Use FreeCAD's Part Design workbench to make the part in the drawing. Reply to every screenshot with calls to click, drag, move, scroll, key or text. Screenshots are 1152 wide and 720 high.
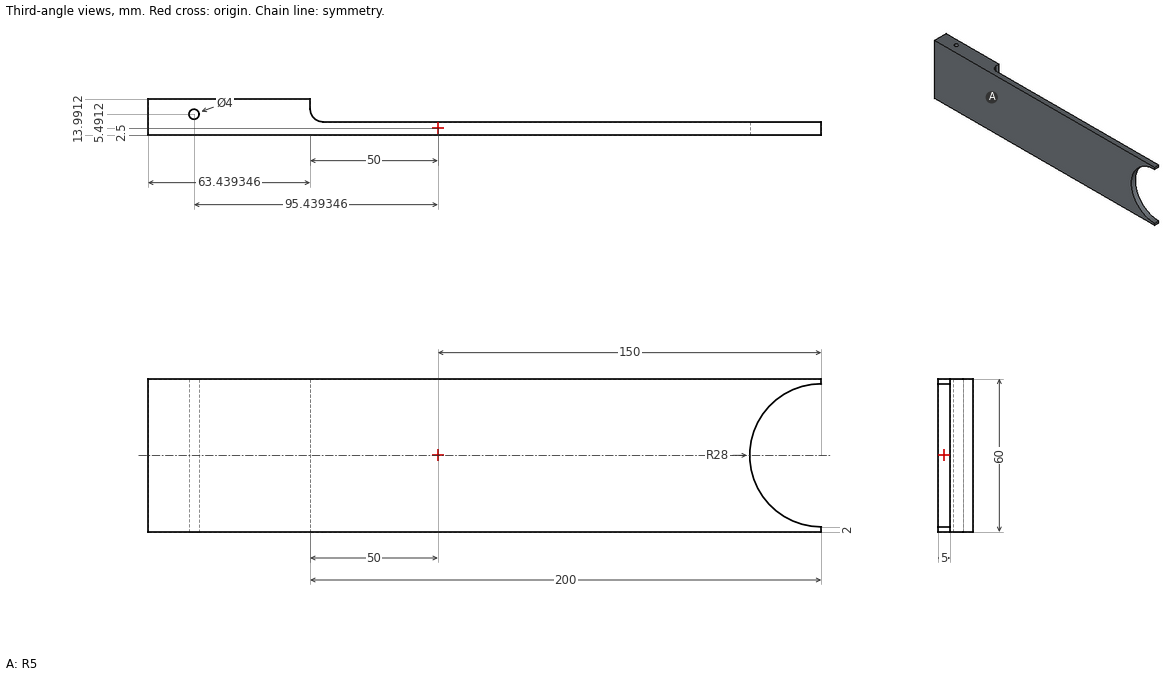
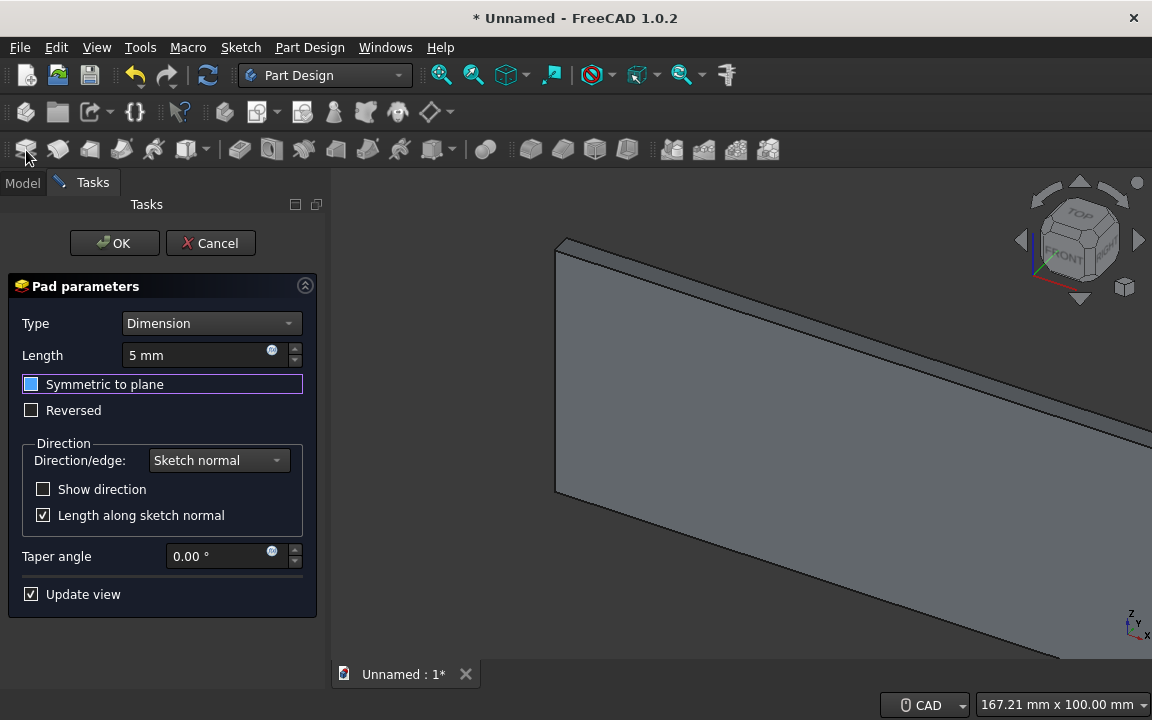
click(30, 384)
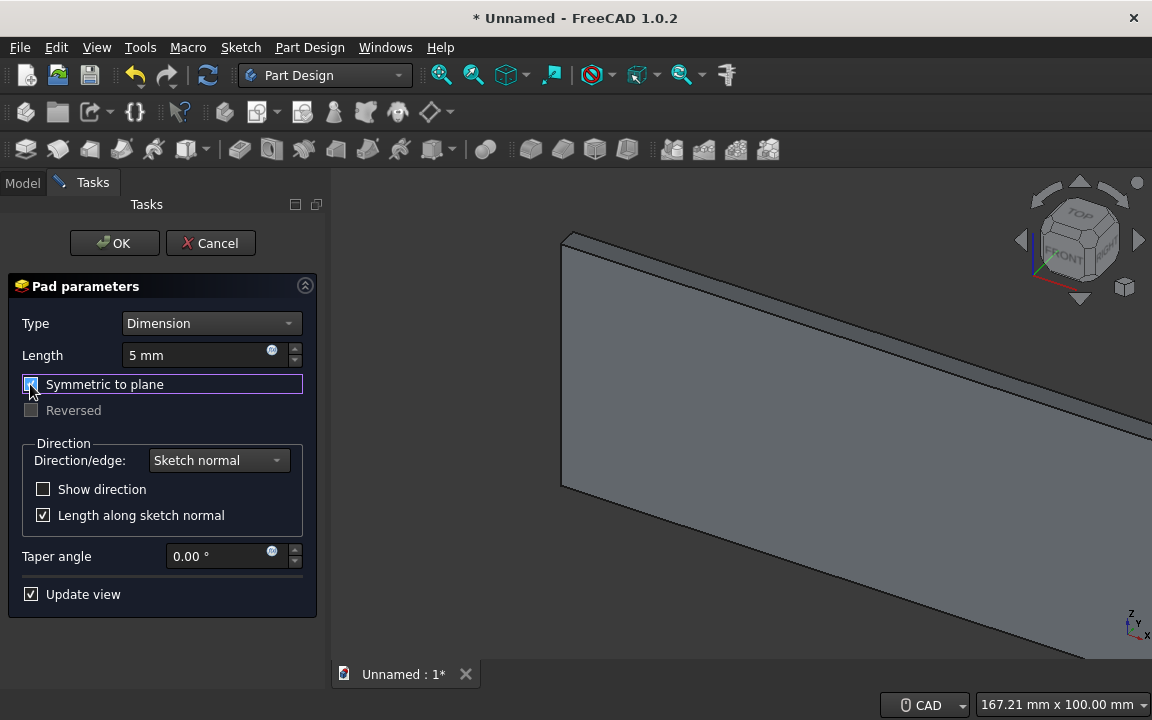
click(115, 243)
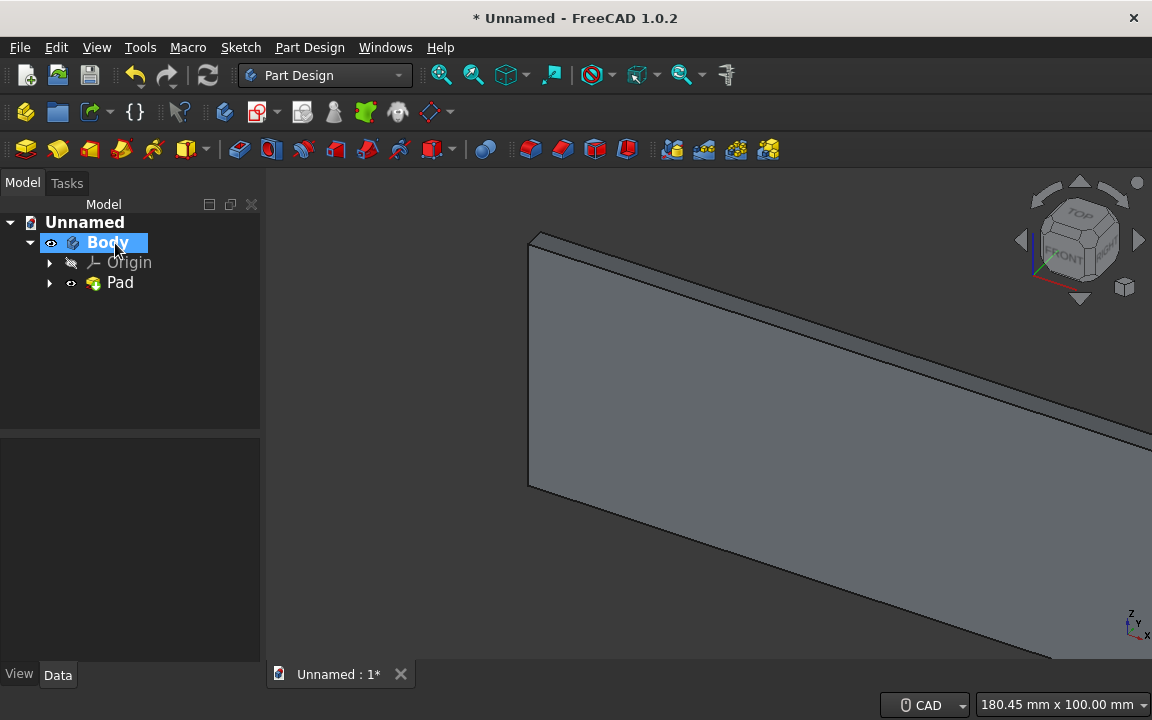
click(442, 76)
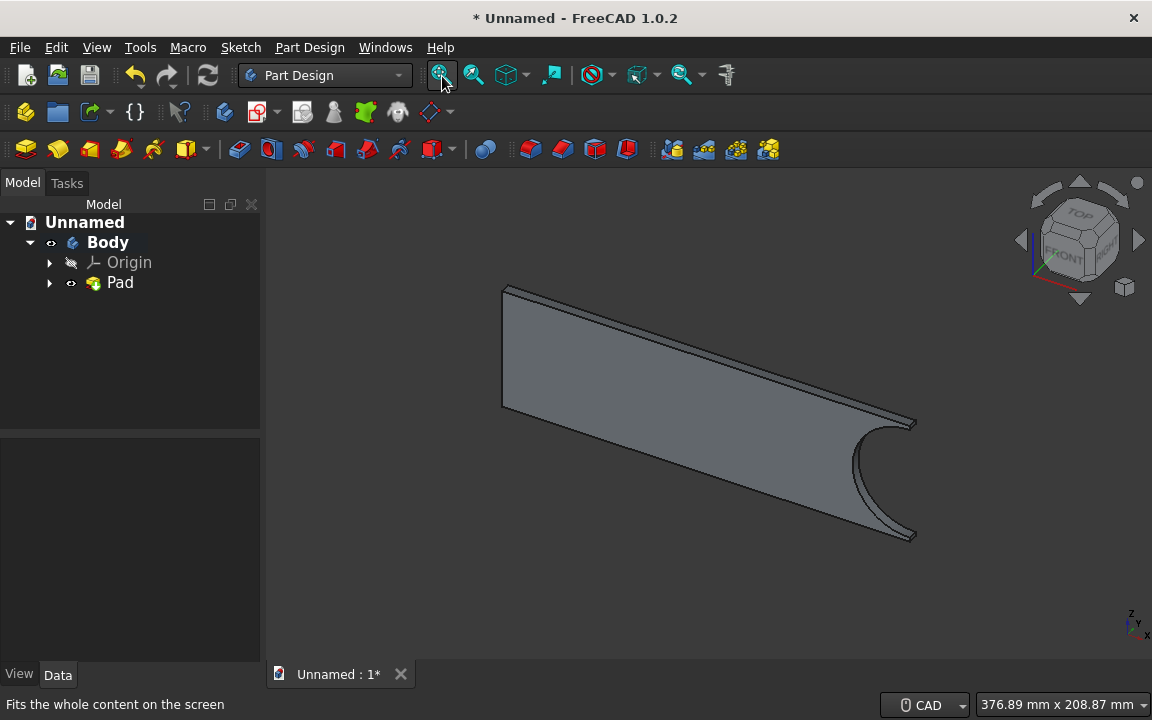
click(258, 112)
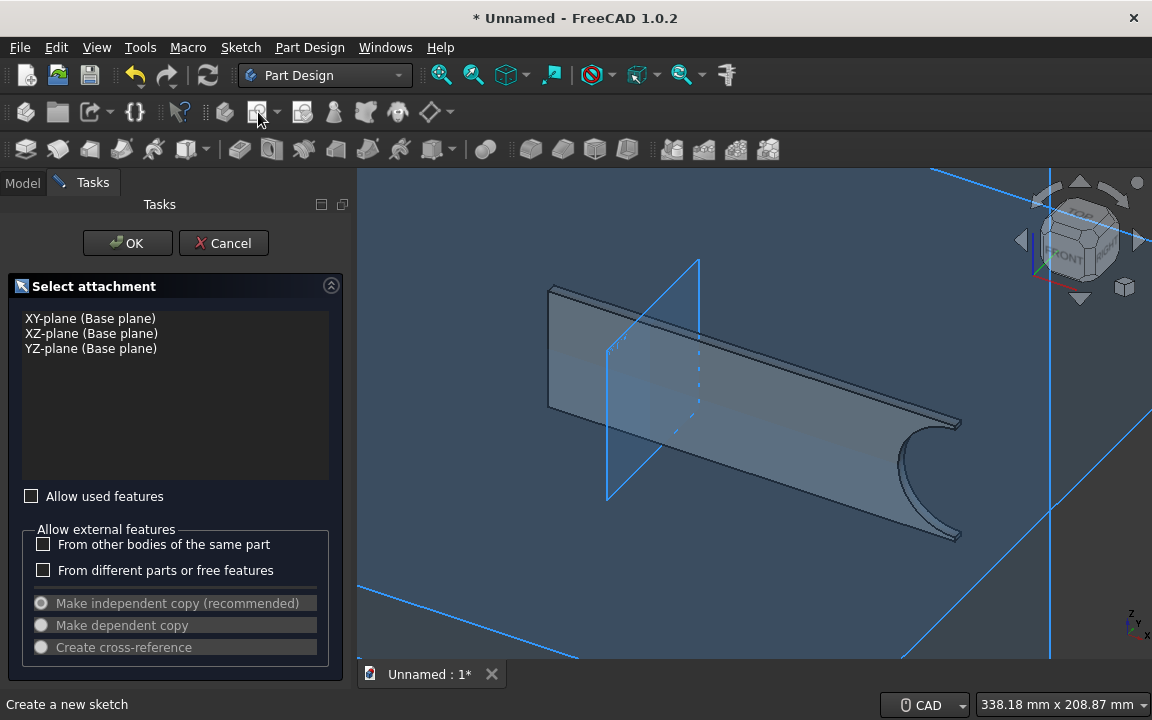
click(82, 318)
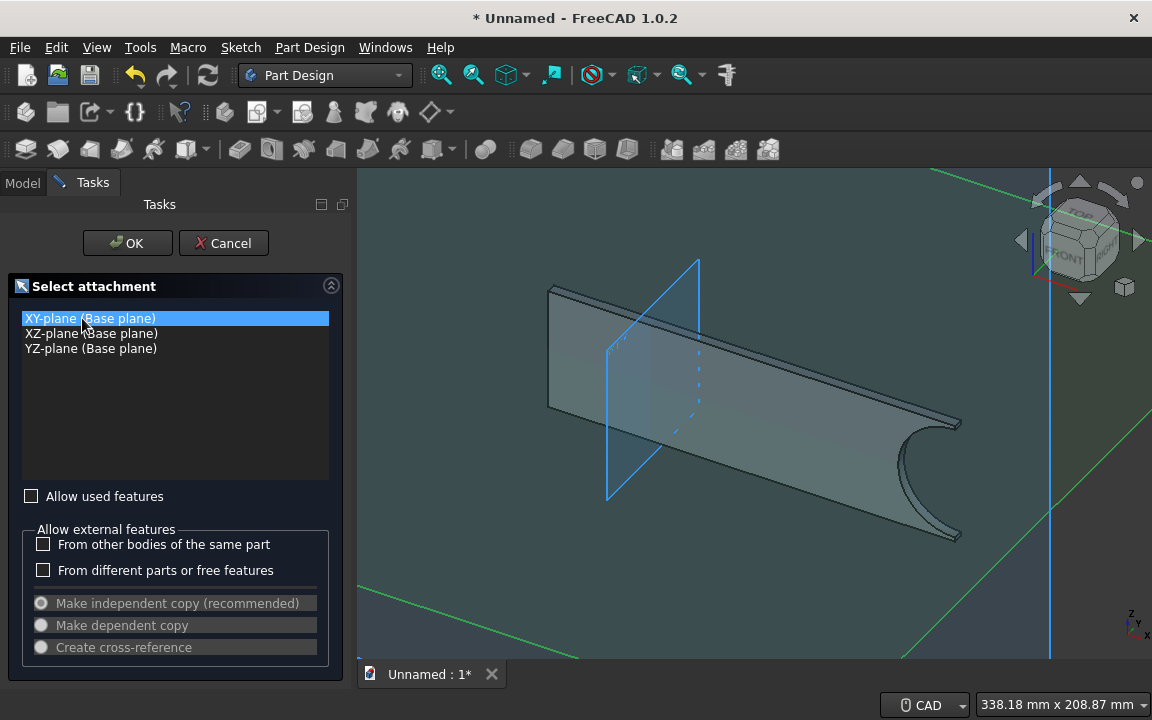
click(128, 243)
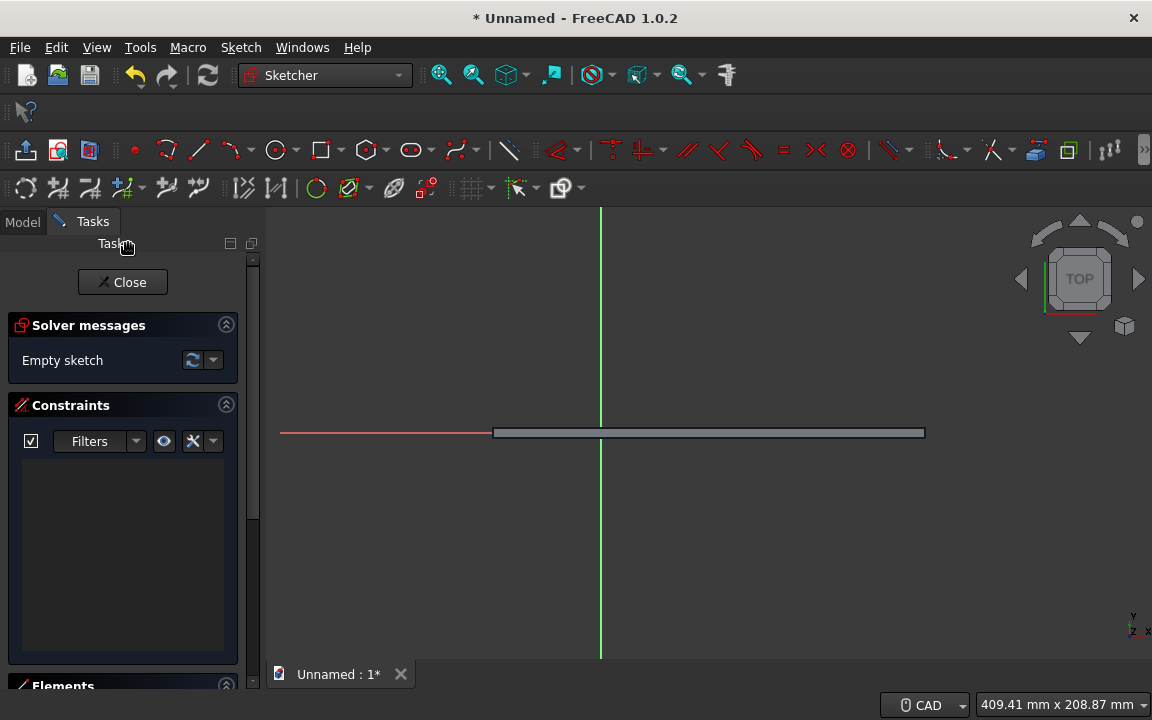
click(90, 150)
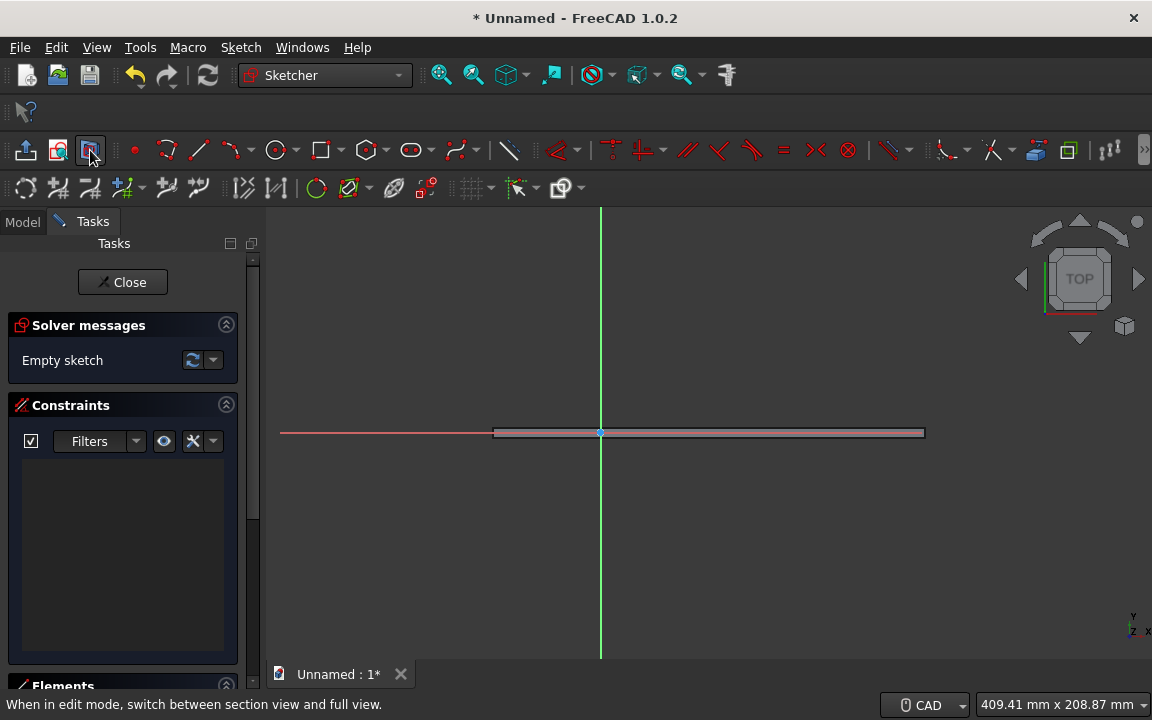
scroll(294, 411, up, 3)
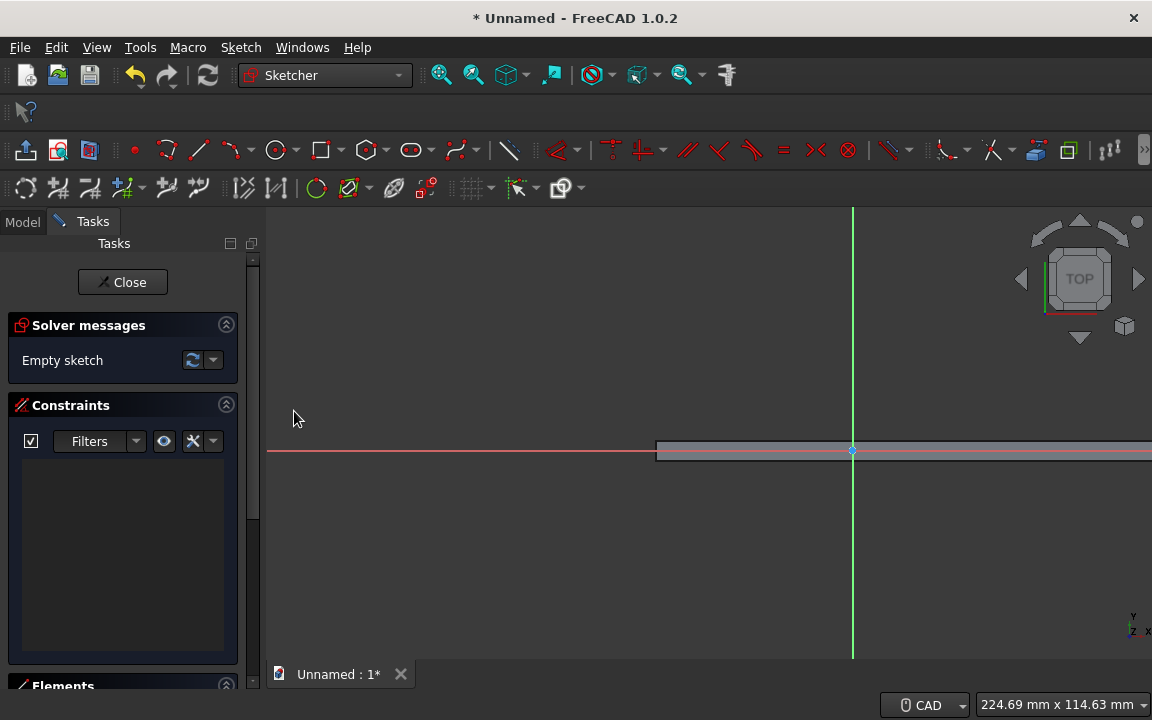
click(322, 150)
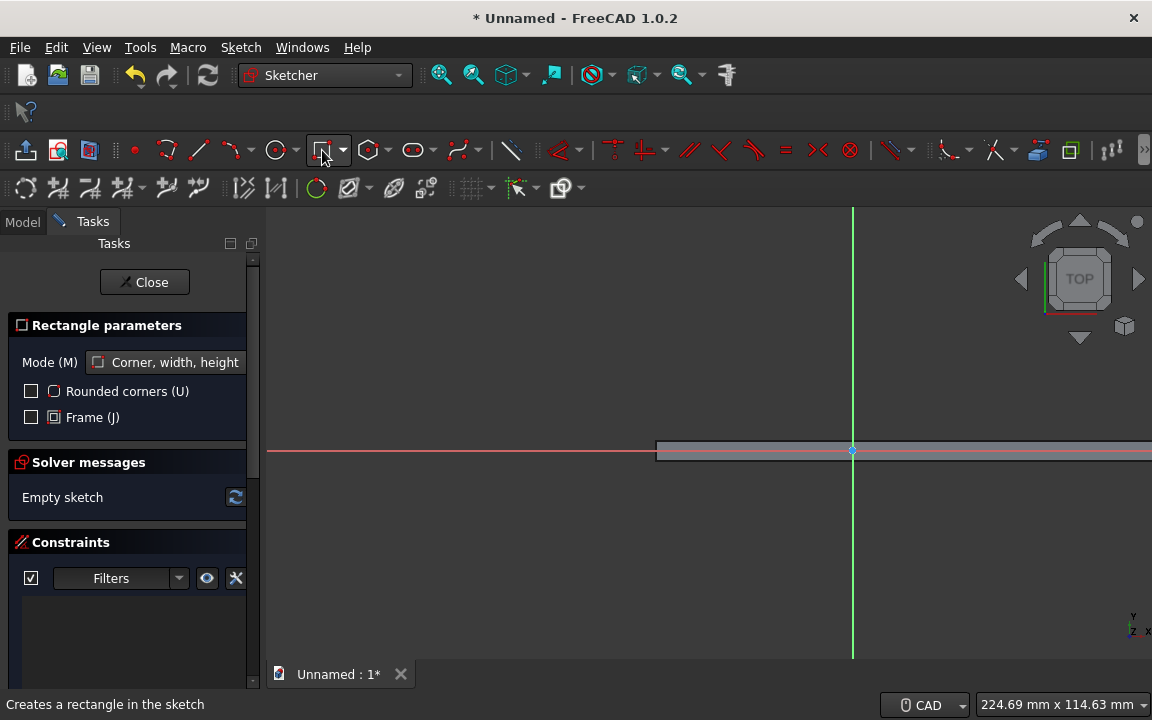
click(406, 405)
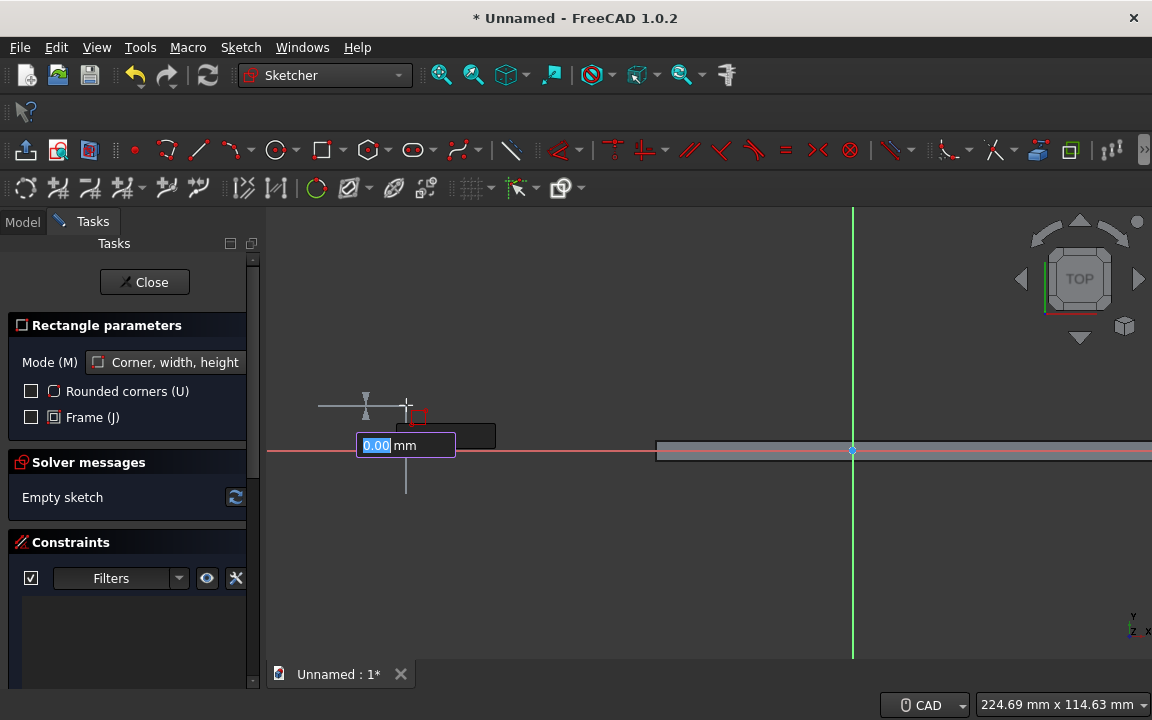
scroll(656, 461, up, 3)
move(655, 460)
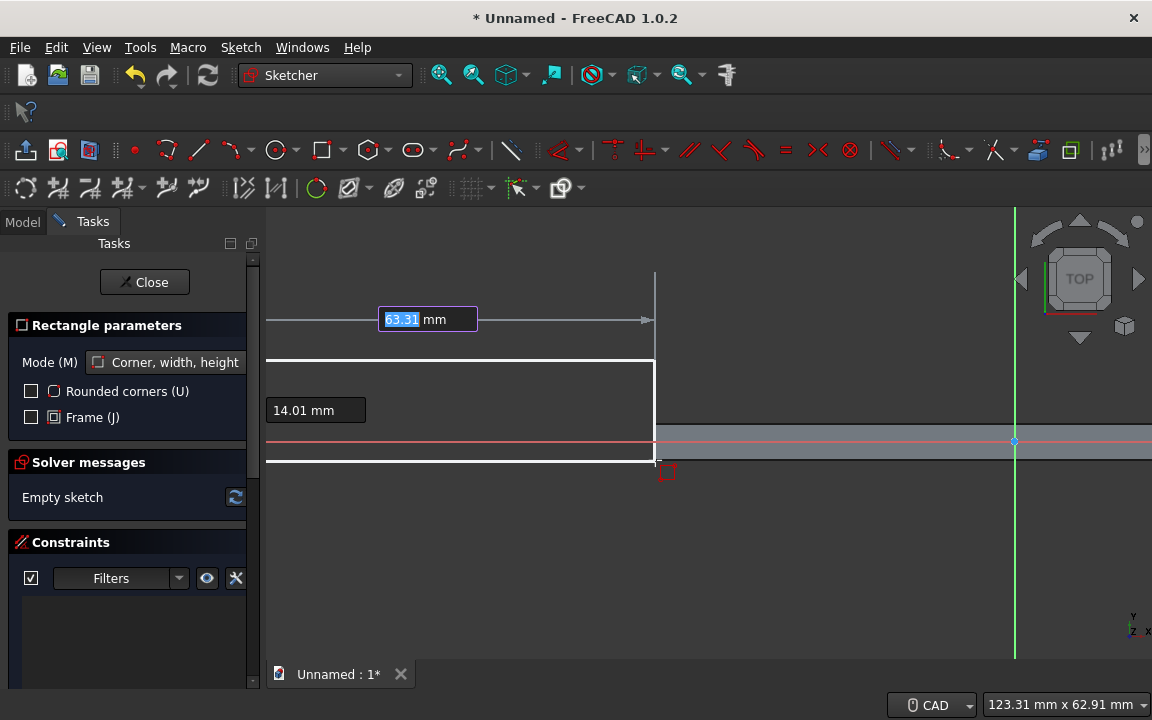
text(63.439346)
key(Tab)
text(13.9912)
key(Return)
key(Escape)